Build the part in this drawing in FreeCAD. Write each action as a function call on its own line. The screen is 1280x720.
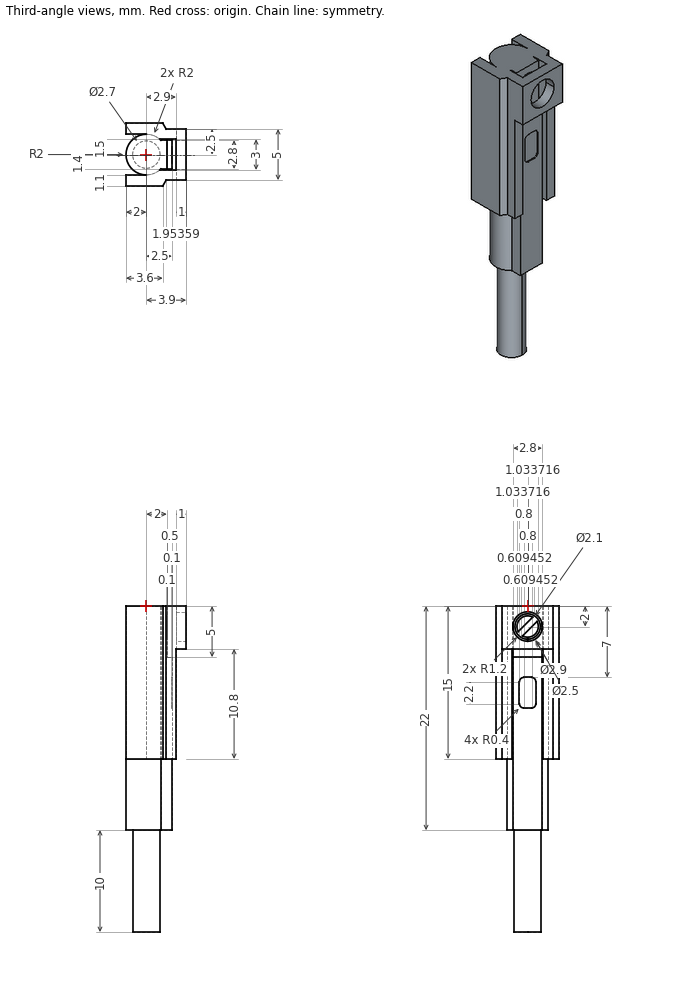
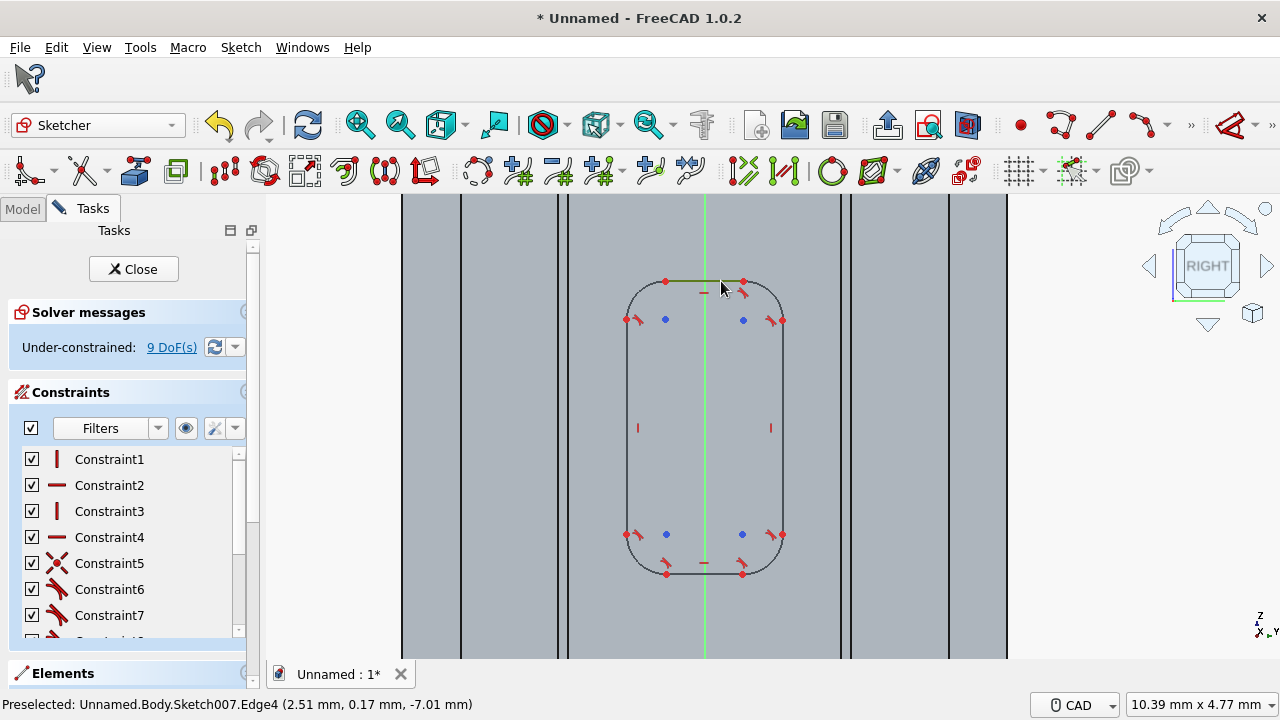
click(648, 285)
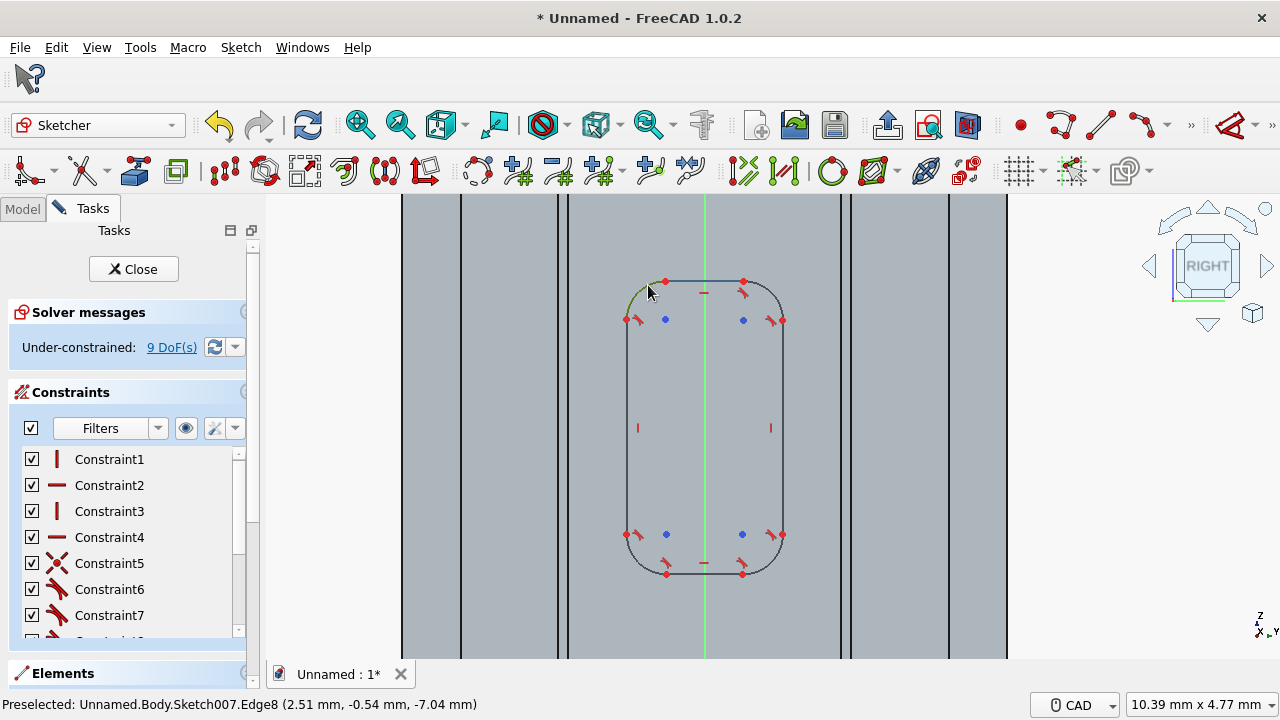
key(t)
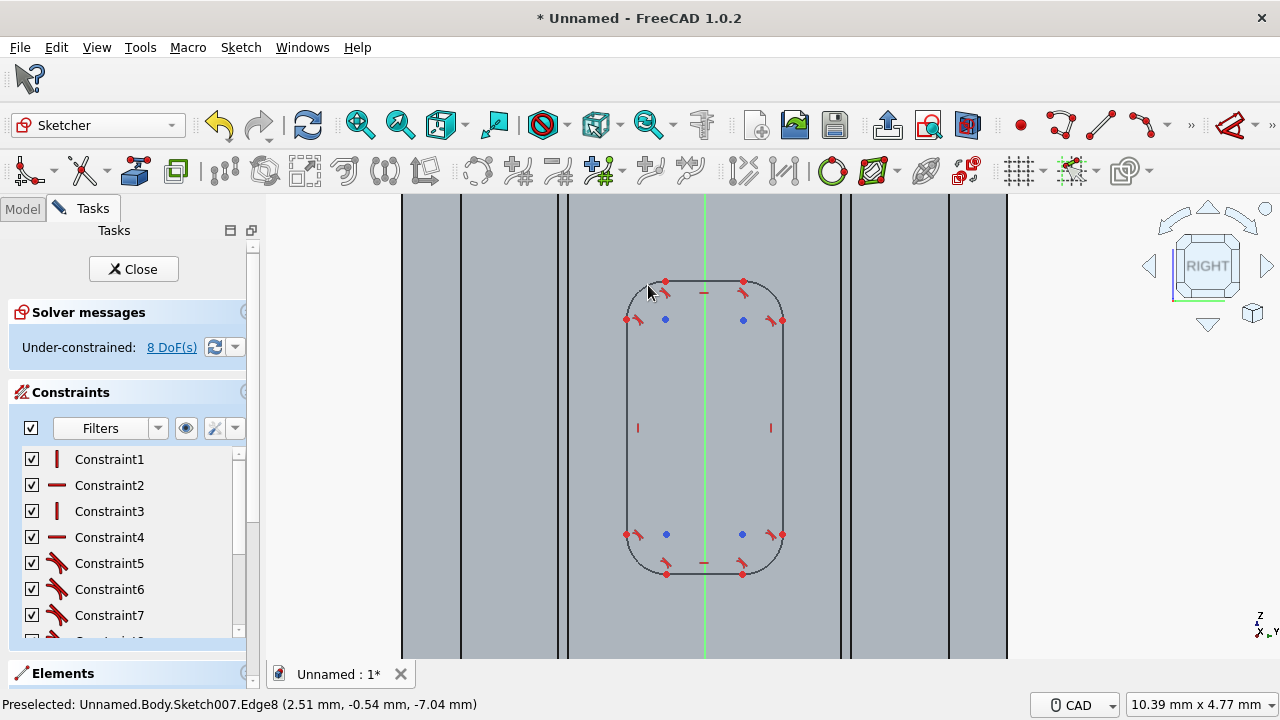
click(631, 553)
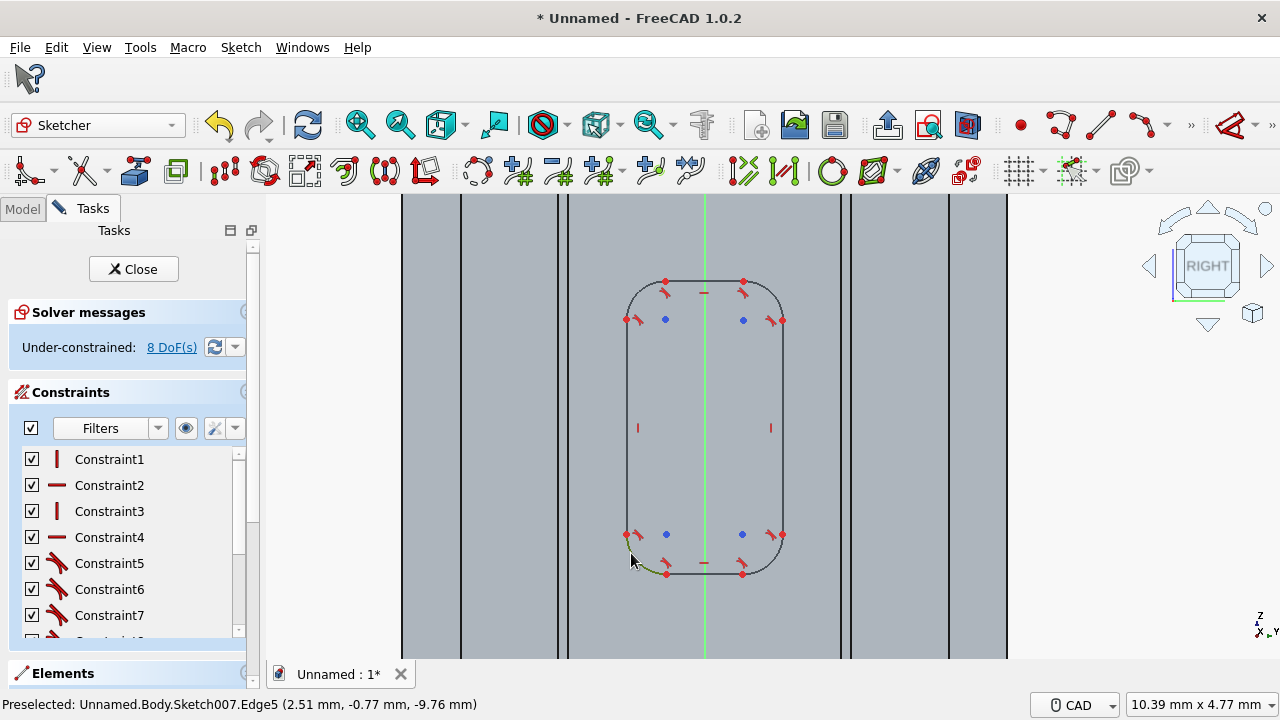
click(761, 570)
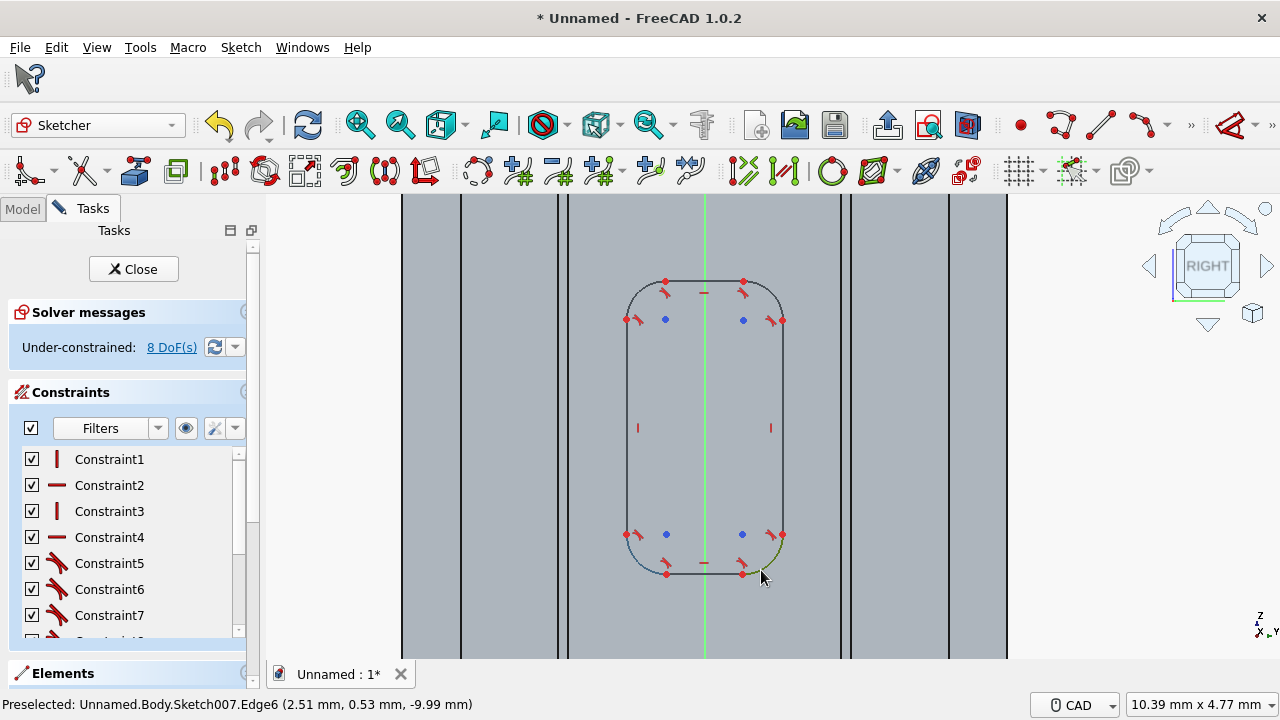
click(779, 303)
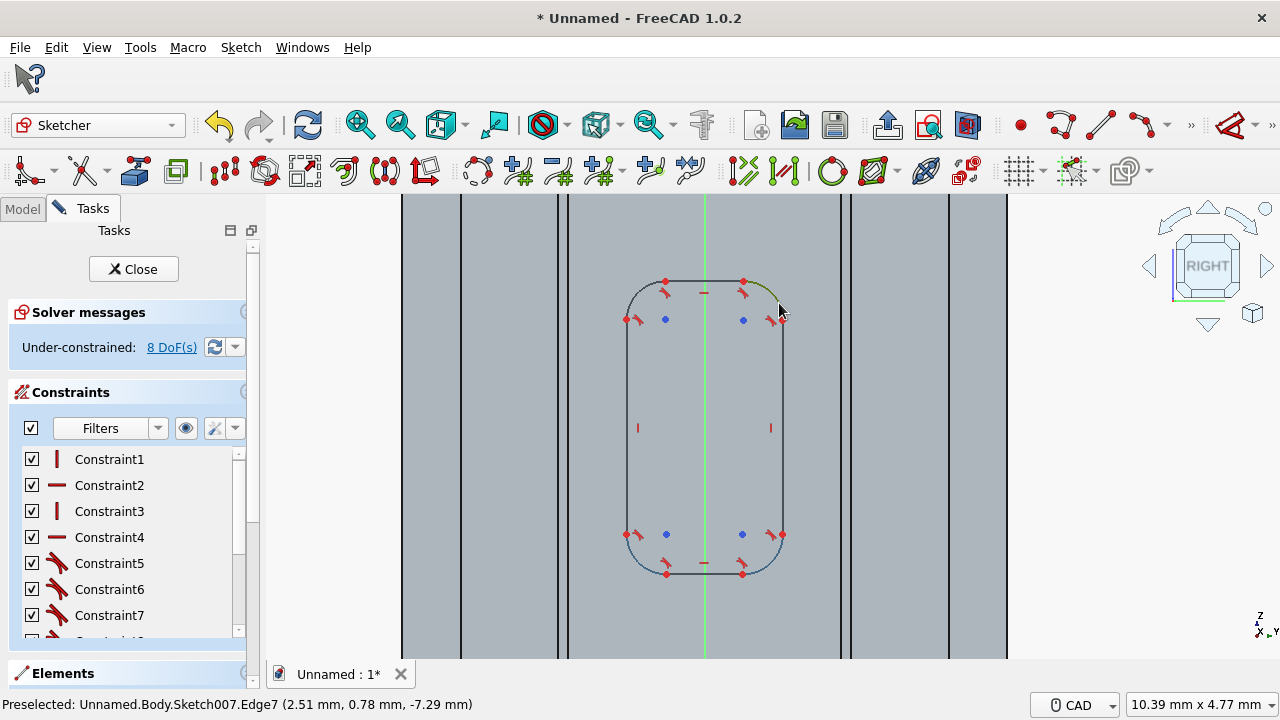
click(648, 286)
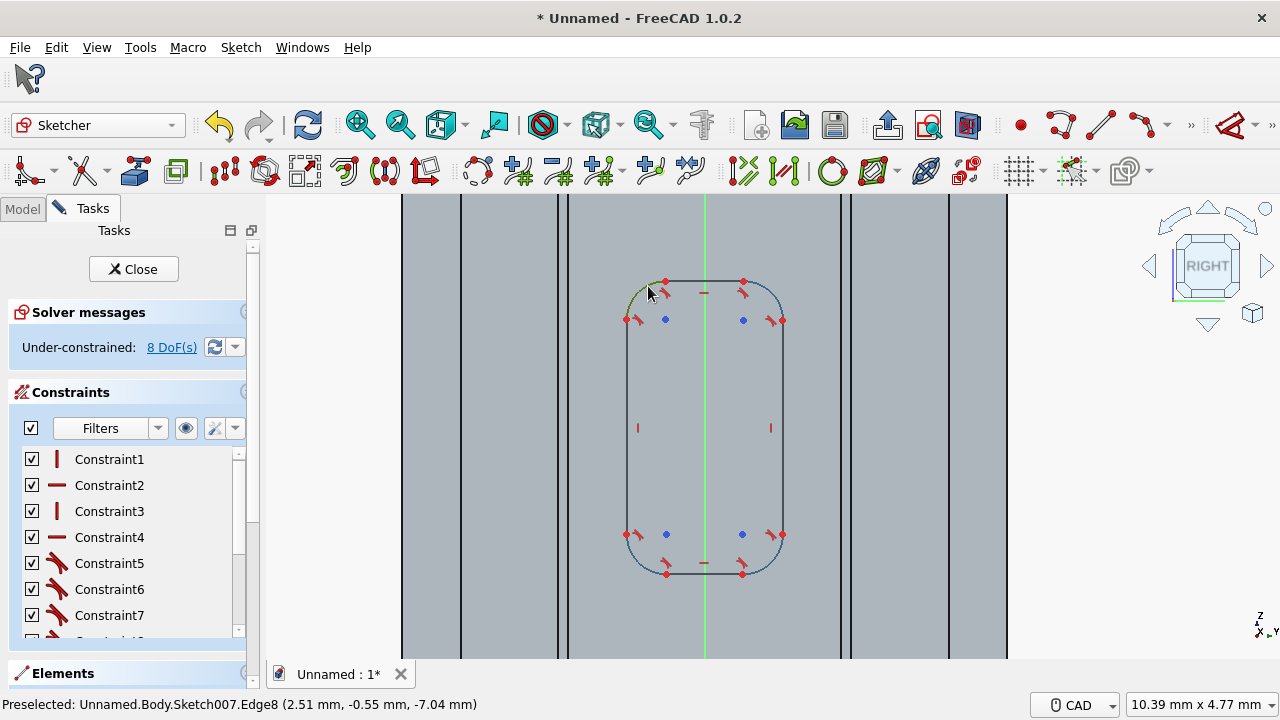
key(e)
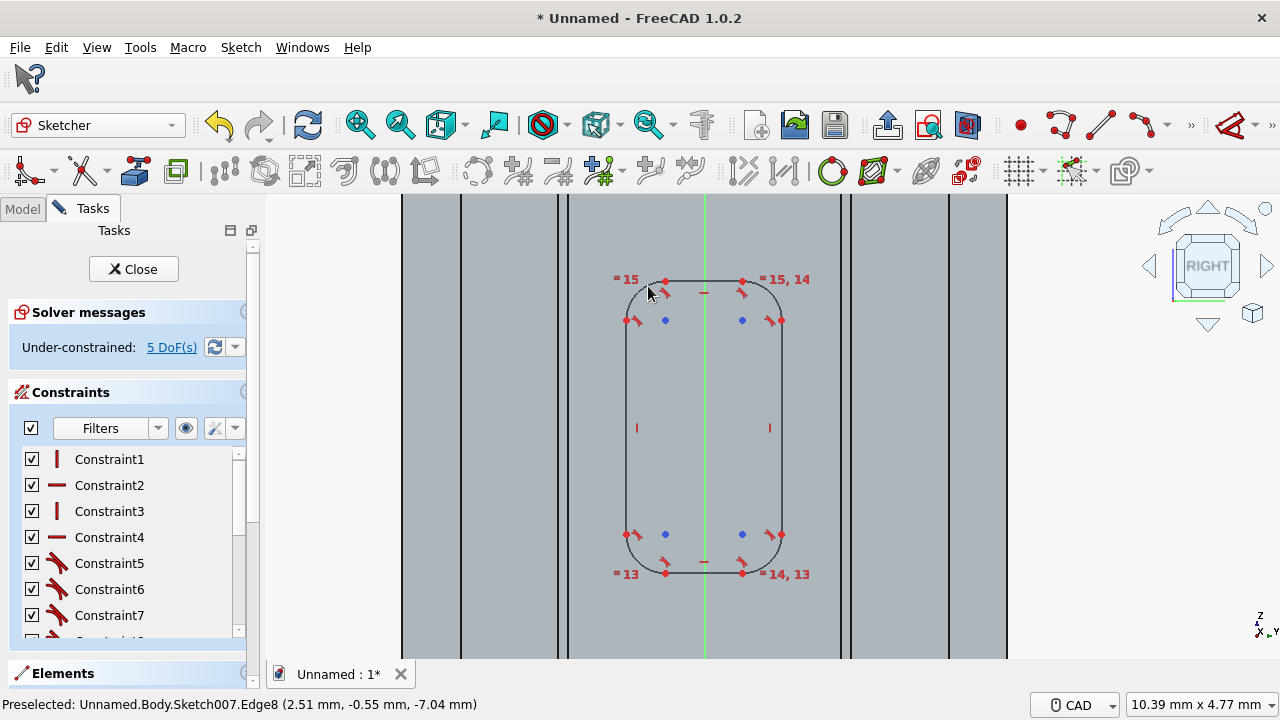
click(1230, 126)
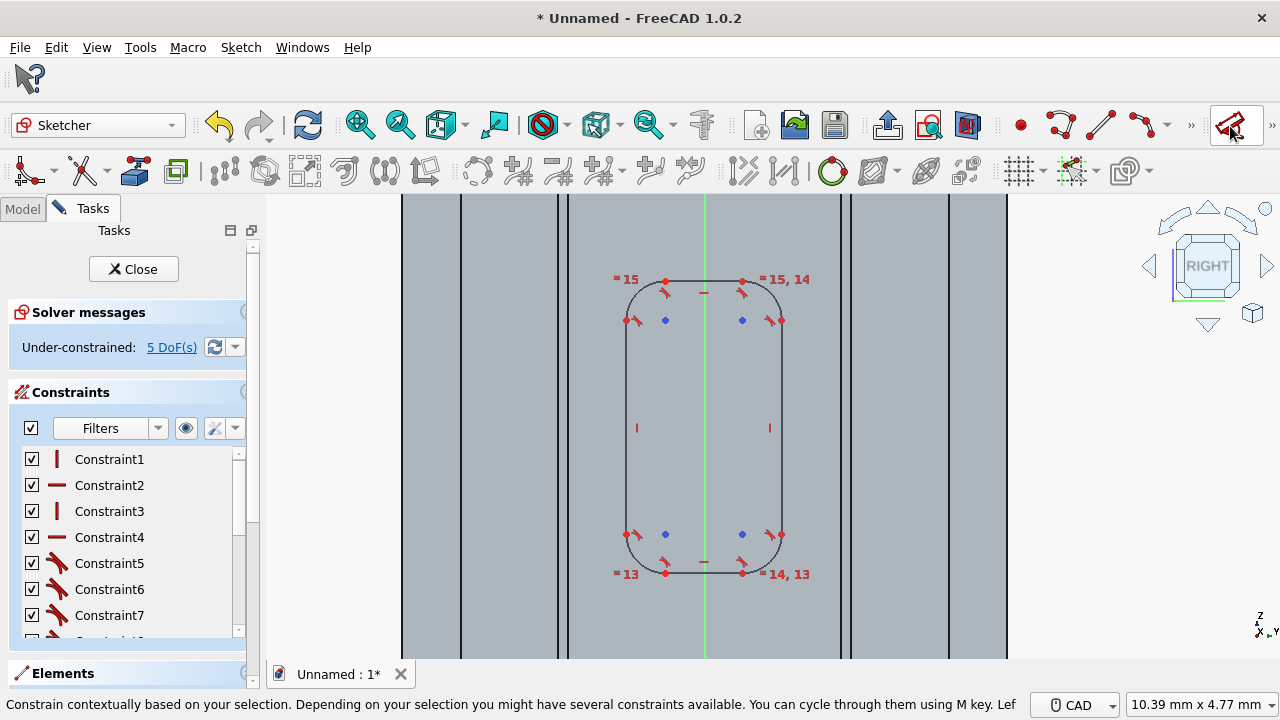
click(631, 552)
click(603, 567)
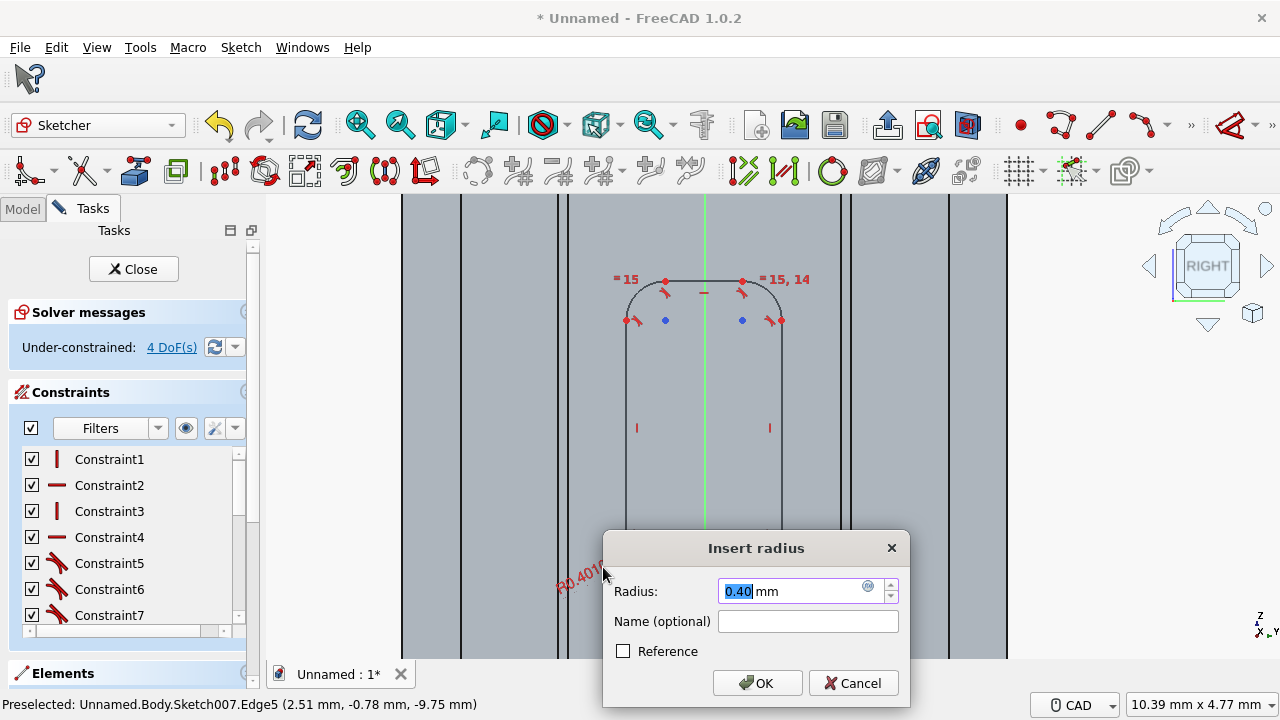
text(0.4)
key(Return)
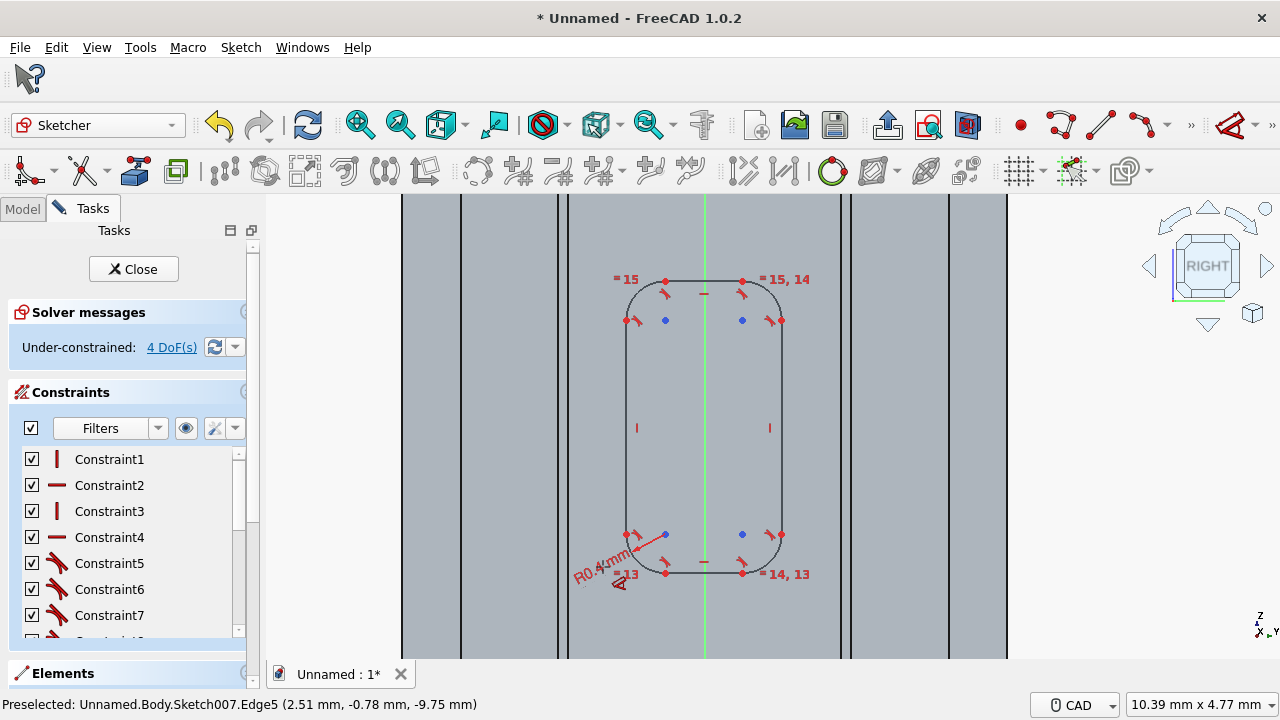
click(743, 281)
click(777, 252)